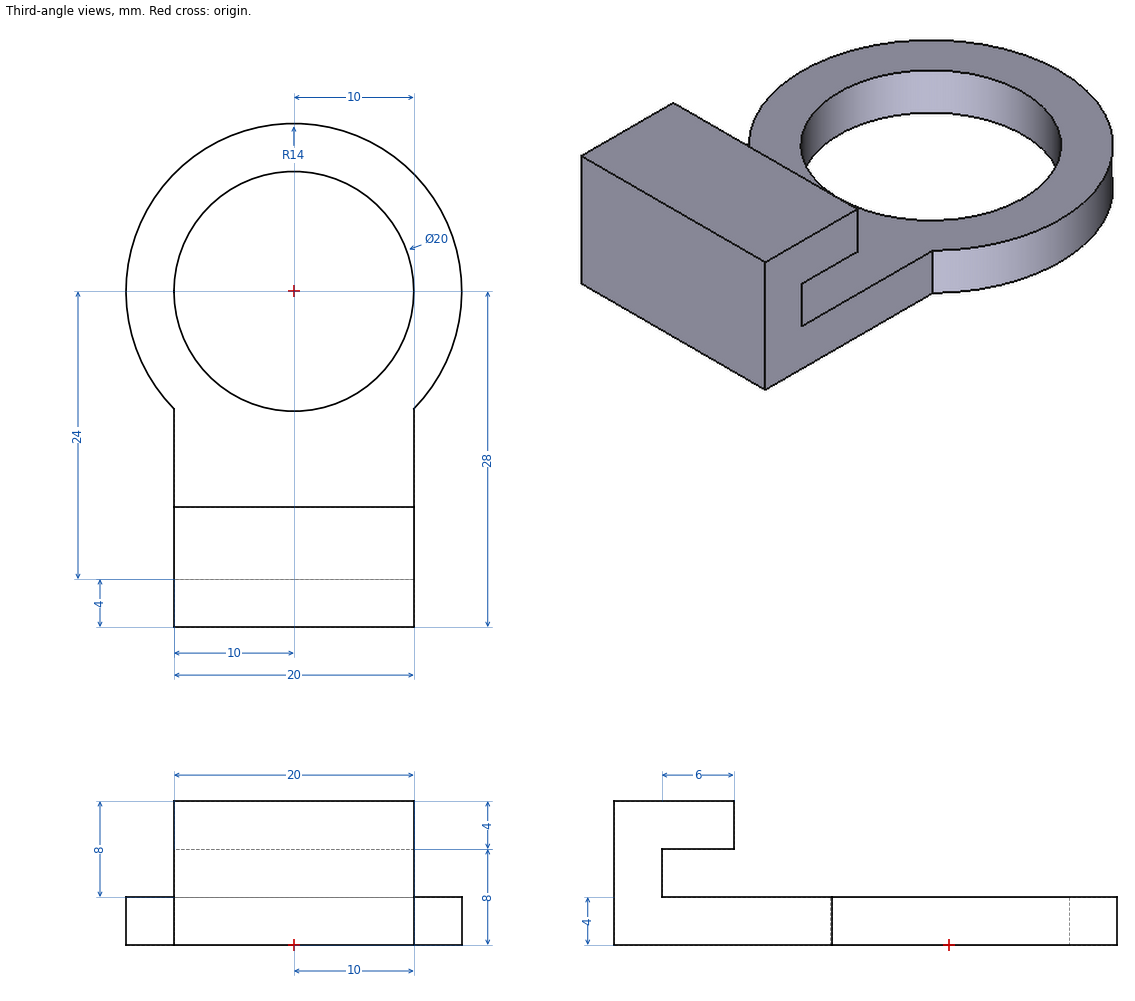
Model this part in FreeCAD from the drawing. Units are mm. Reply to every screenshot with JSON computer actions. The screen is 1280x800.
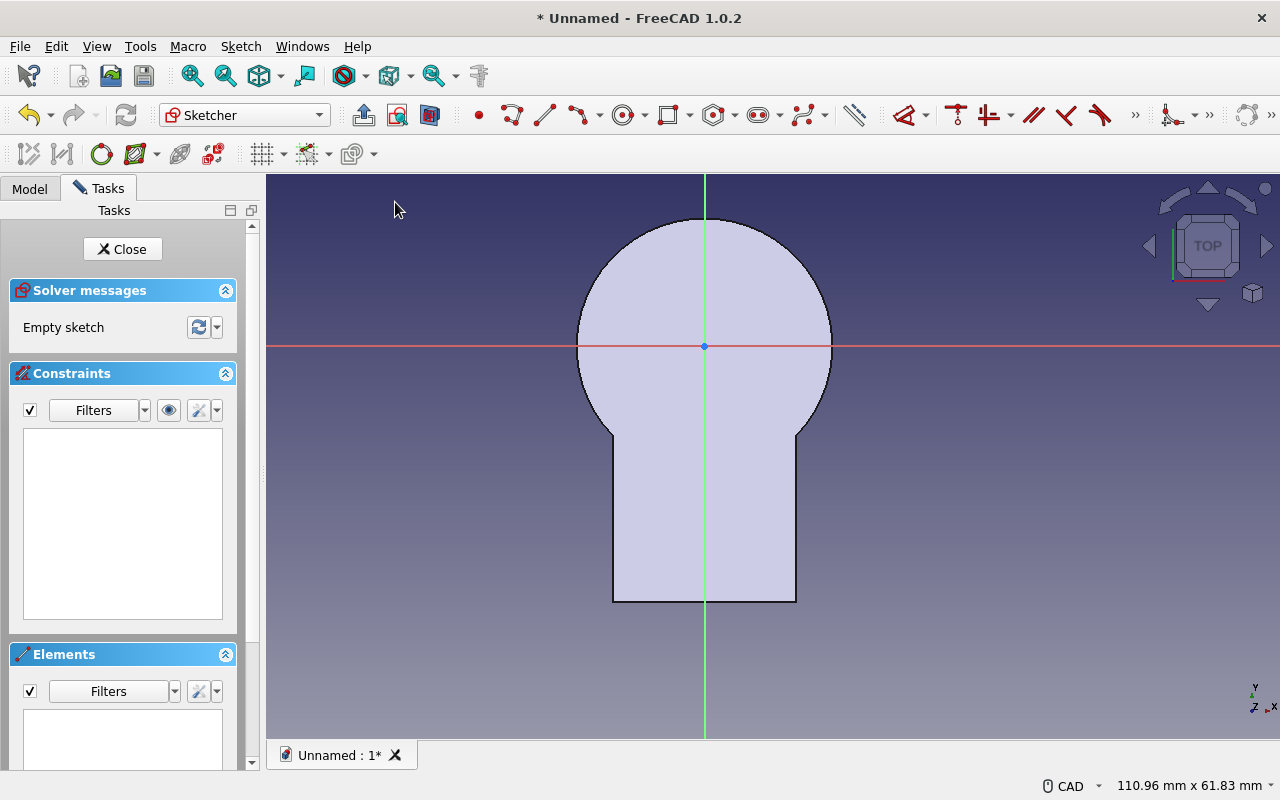
{"action": "scroll", "coordinate": [705, 511], "scroll_direction": "up", "scroll_amount": 2}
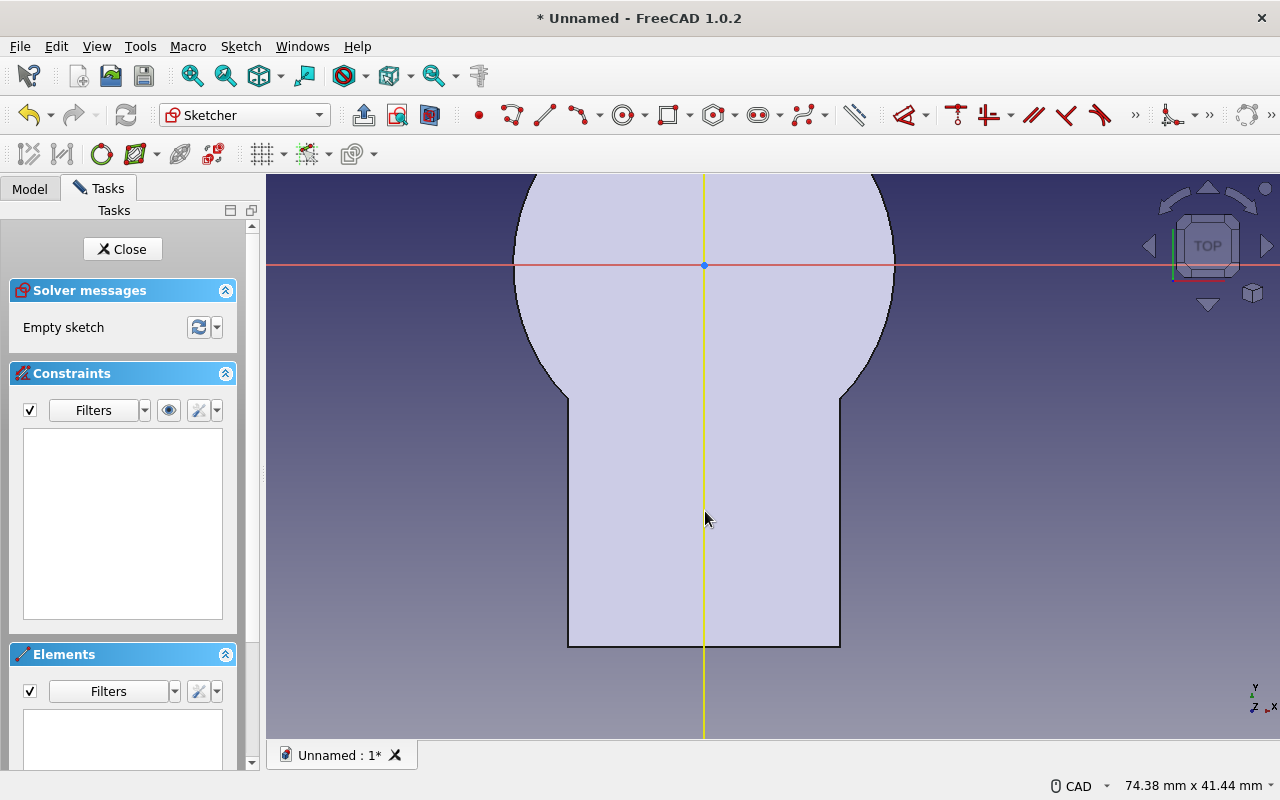
{"action": "key", "text": "g r"}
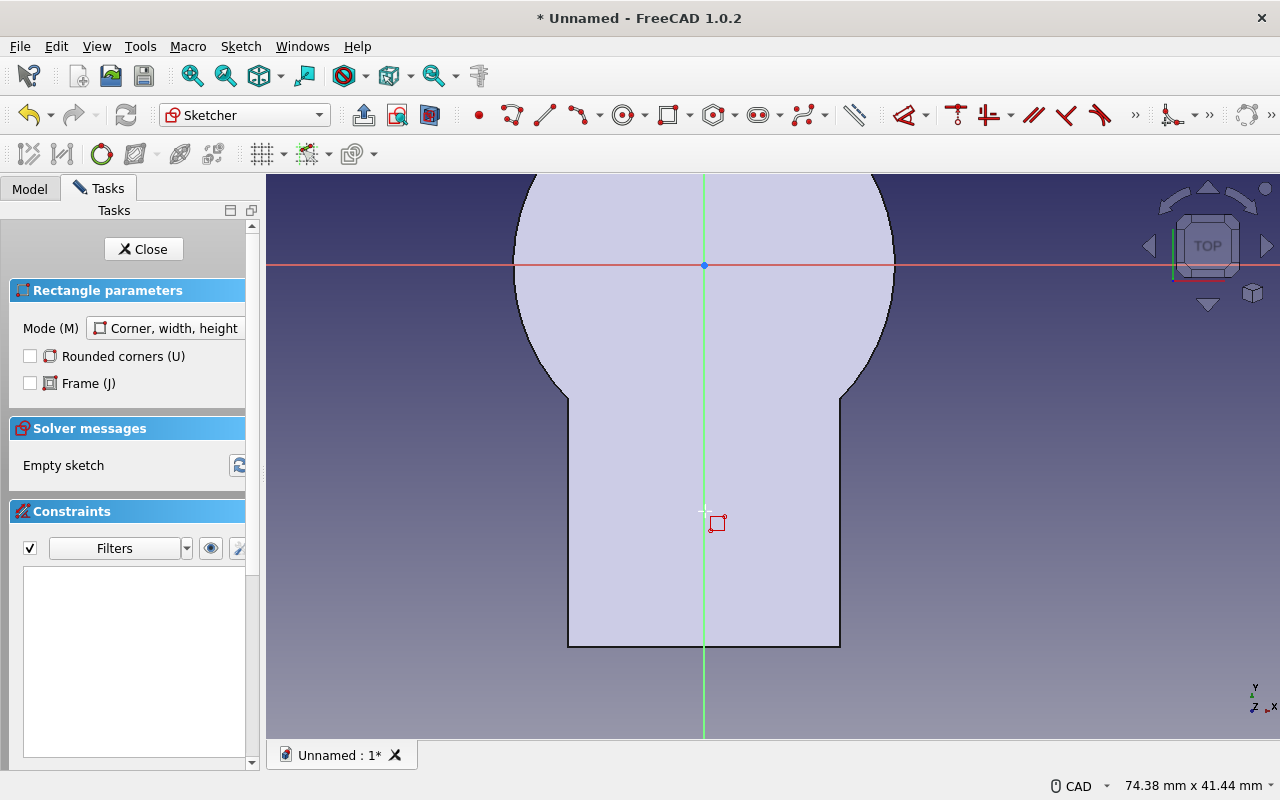
{"action": "left_click", "coordinate": [568, 592]}
{"action": "left_click", "coordinate": [840, 647]}
{"action": "key", "text": "Escape"}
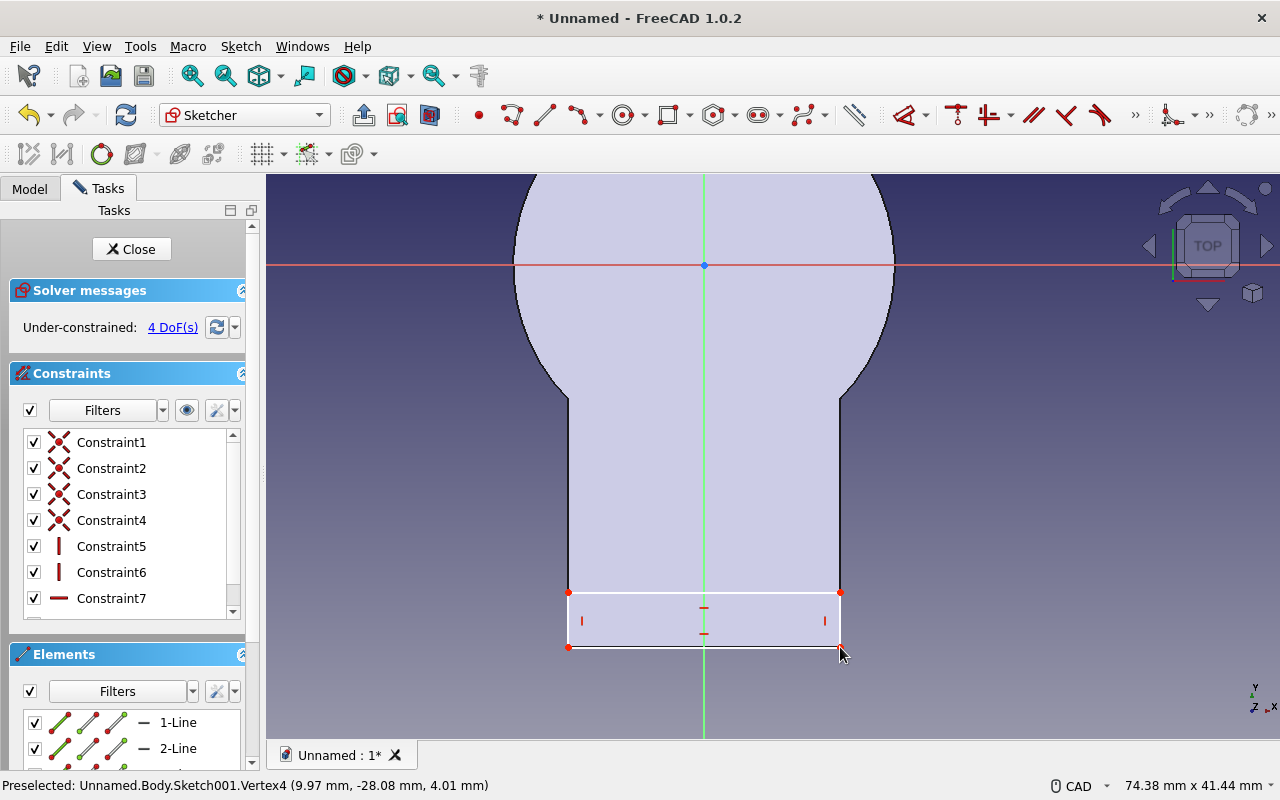
{"action": "left_click", "coordinate": [904, 116]}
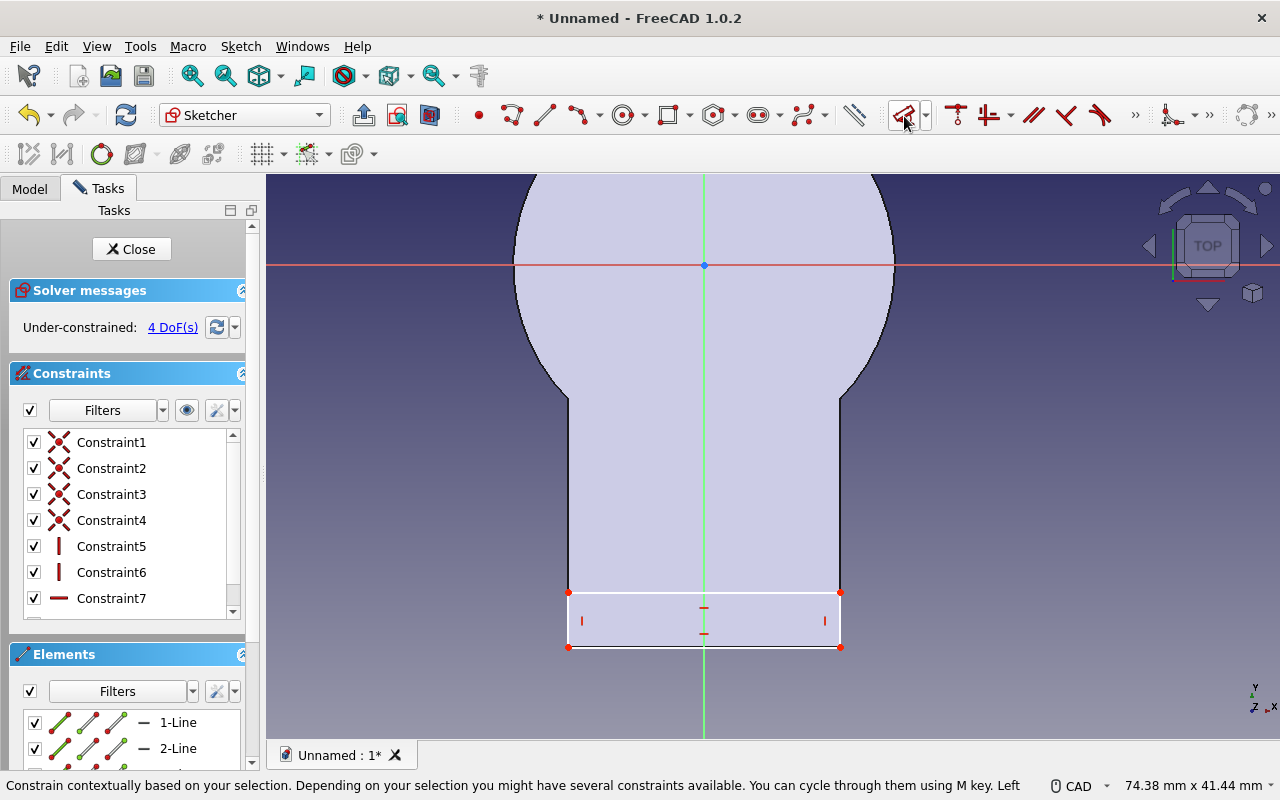
{"action": "left_click", "coordinate": [568, 609]}
{"action": "left_click", "coordinate": [534, 620]}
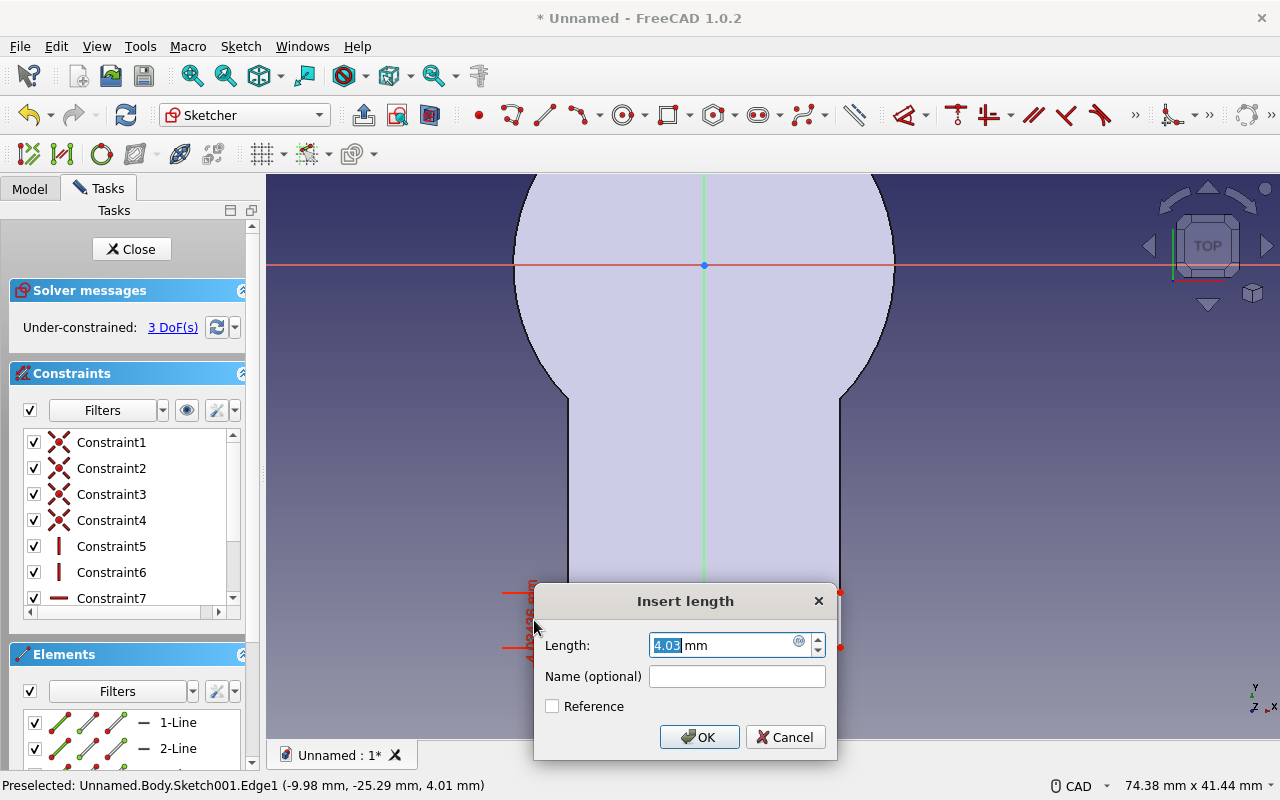
{"action": "type", "text": "4"}
{"action": "key", "text": "Return"}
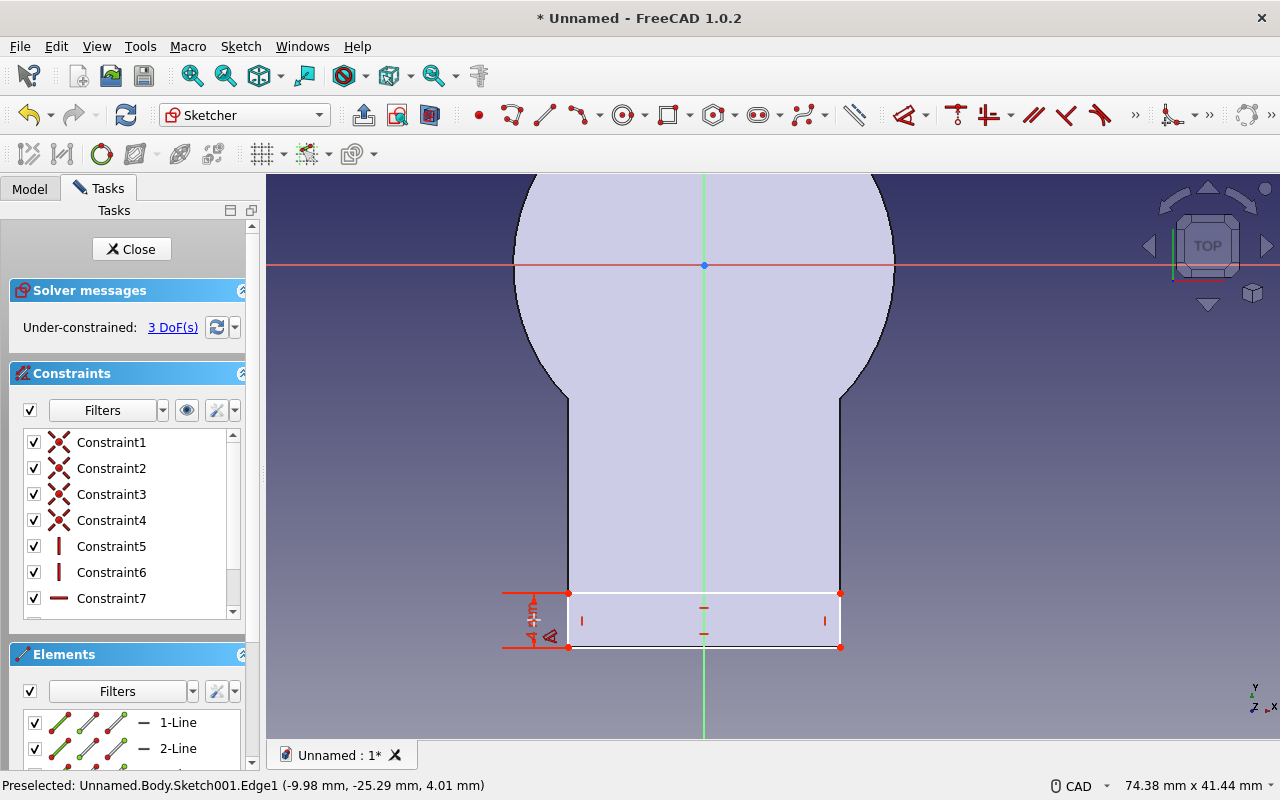
{"action": "left_click", "coordinate": [650, 648]}
{"action": "left_click", "coordinate": [641, 682]}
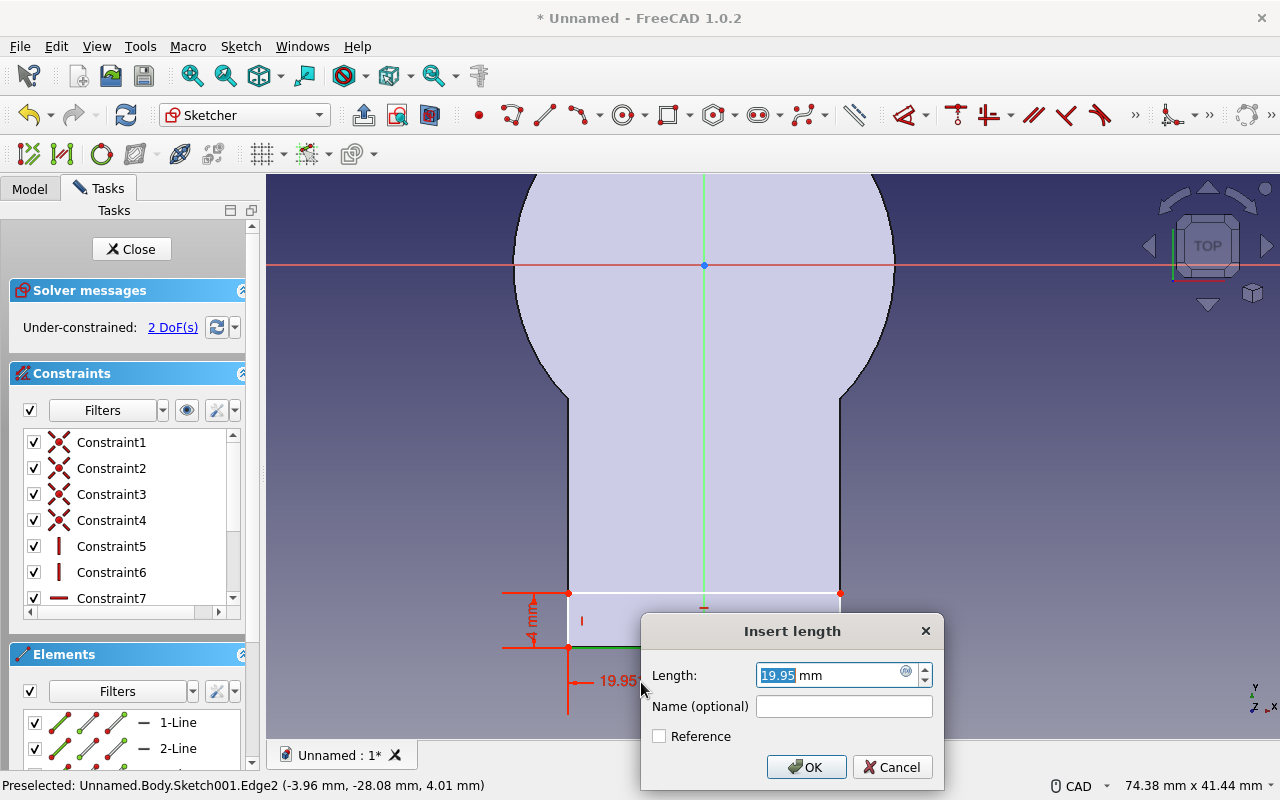
{"action": "type", "text": "20"}
{"action": "key", "text": "Return"}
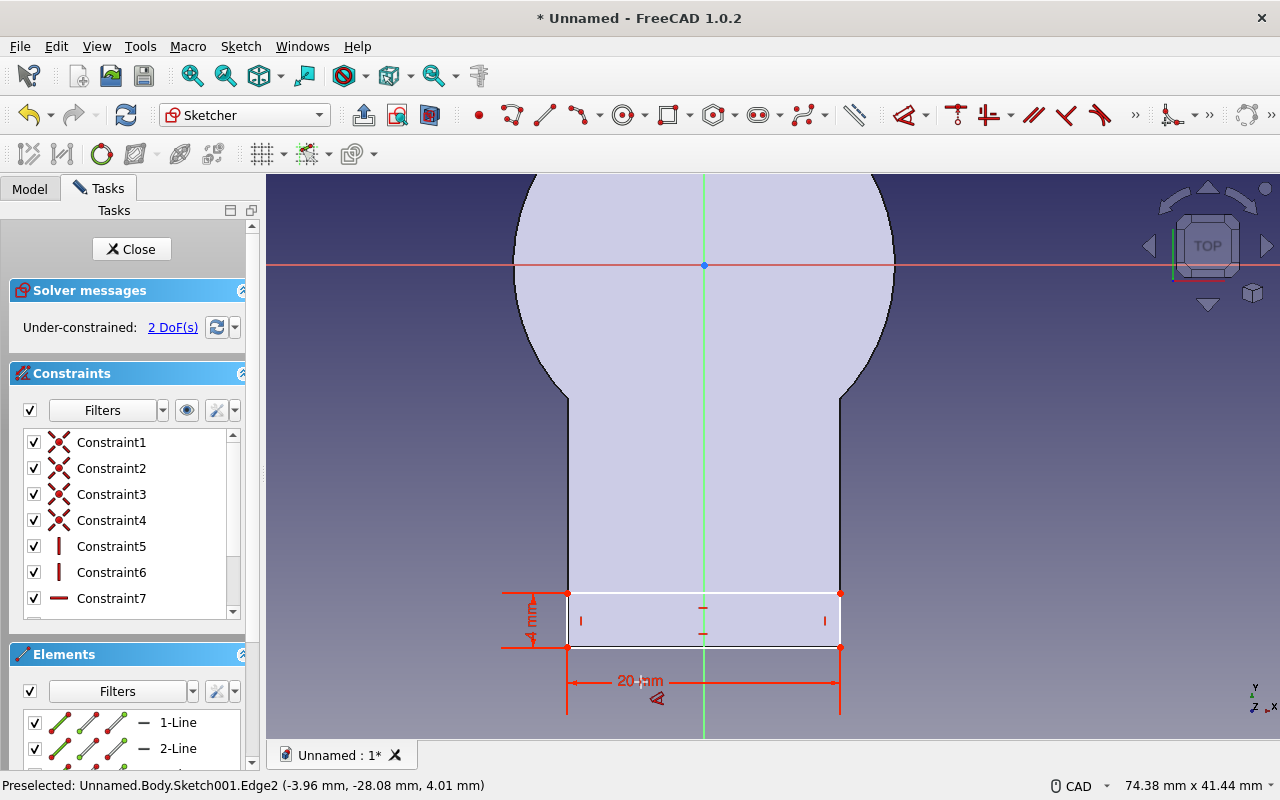
{"action": "left_click", "coordinate": [567, 593]}
{"action": "left_click", "coordinate": [636, 231]}